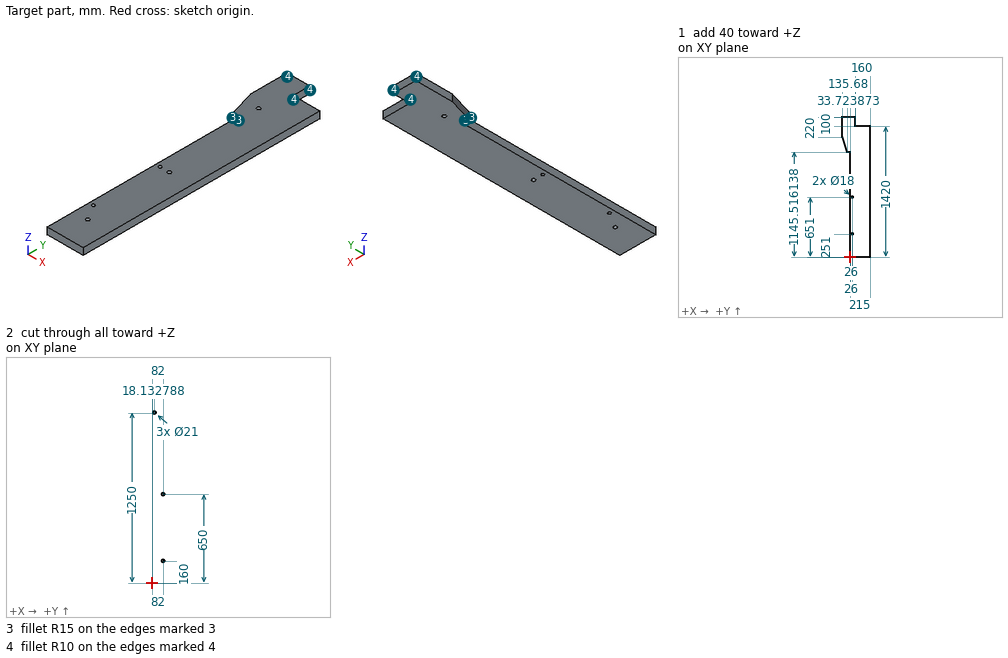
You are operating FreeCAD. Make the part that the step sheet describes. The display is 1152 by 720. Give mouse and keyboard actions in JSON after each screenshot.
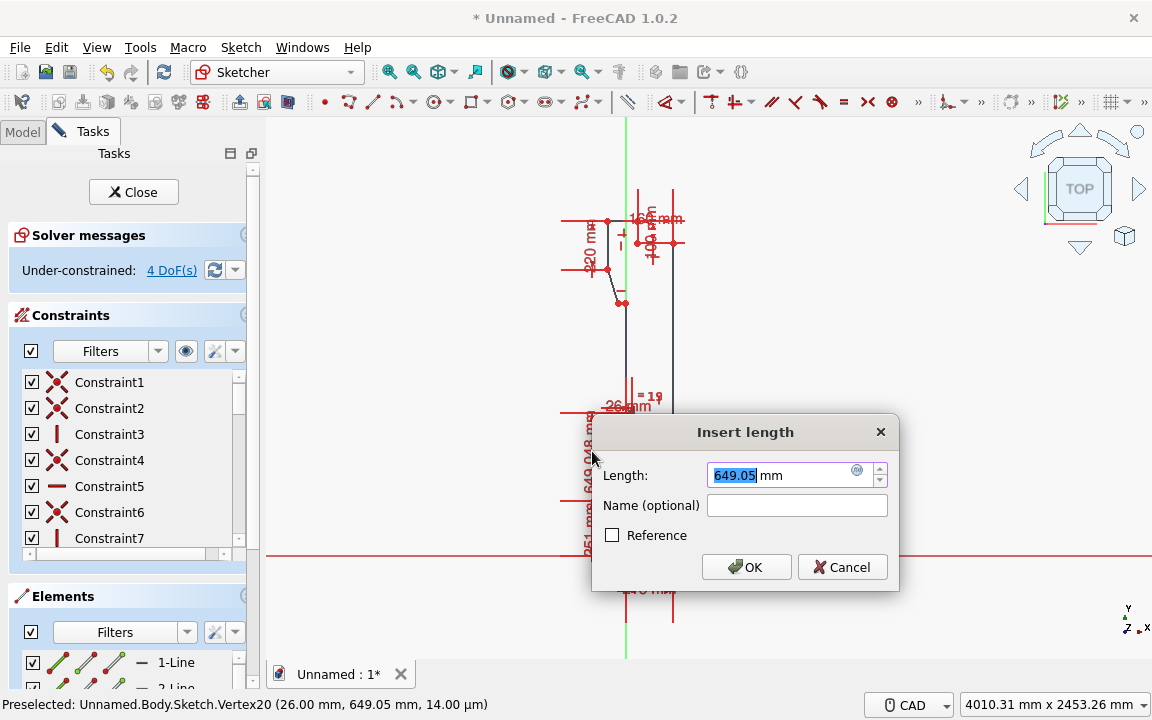
{"action": "type", "text": "651"}
{"action": "key", "text": "Return"}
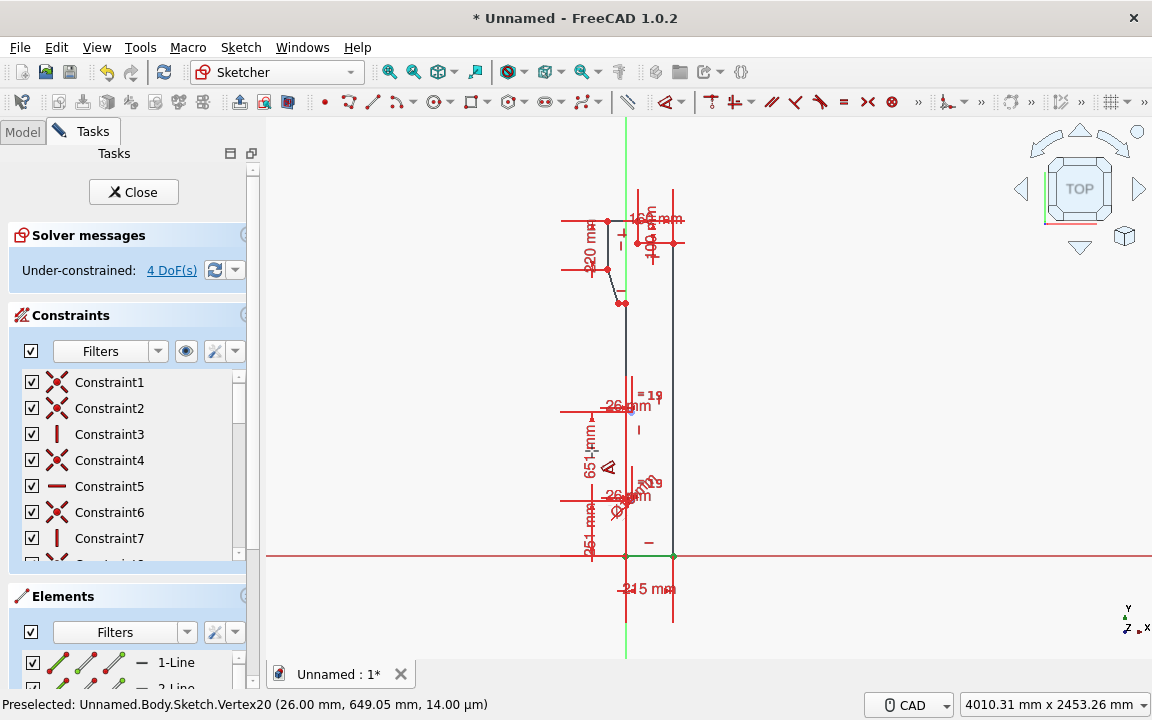
{"action": "left_click", "coordinate": [673, 462]}
{"action": "left_click", "coordinate": [707, 400]}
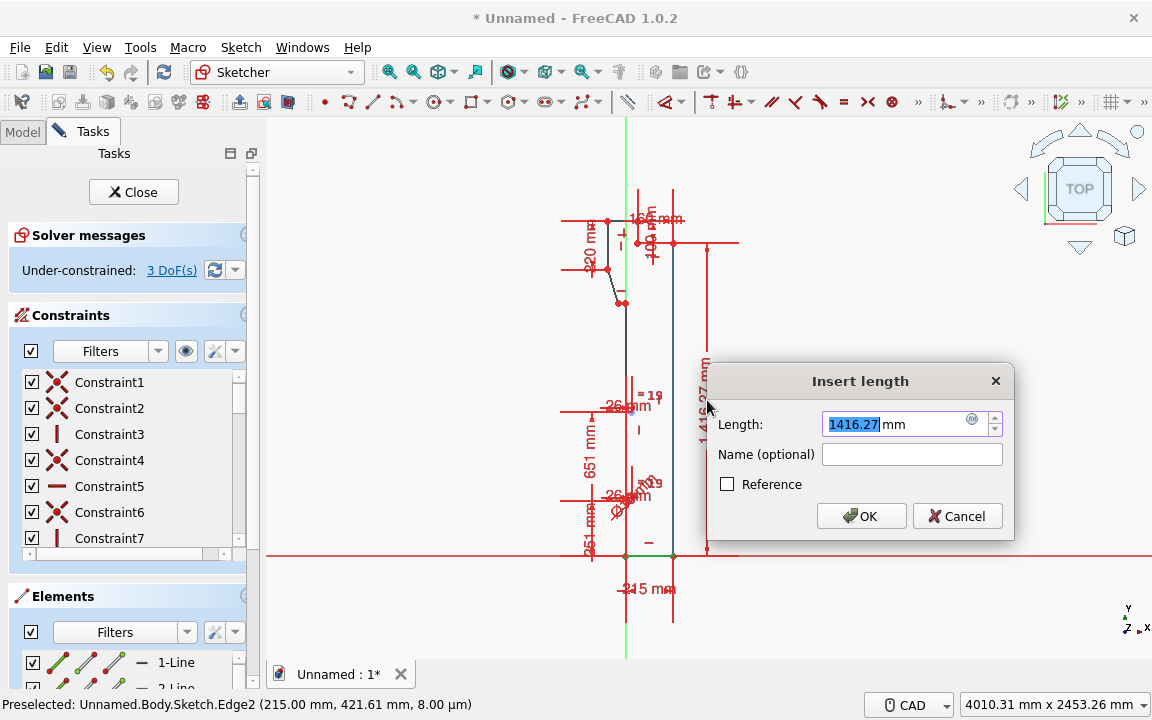
{"action": "type", "text": "1420"}
{"action": "key", "text": "Return"}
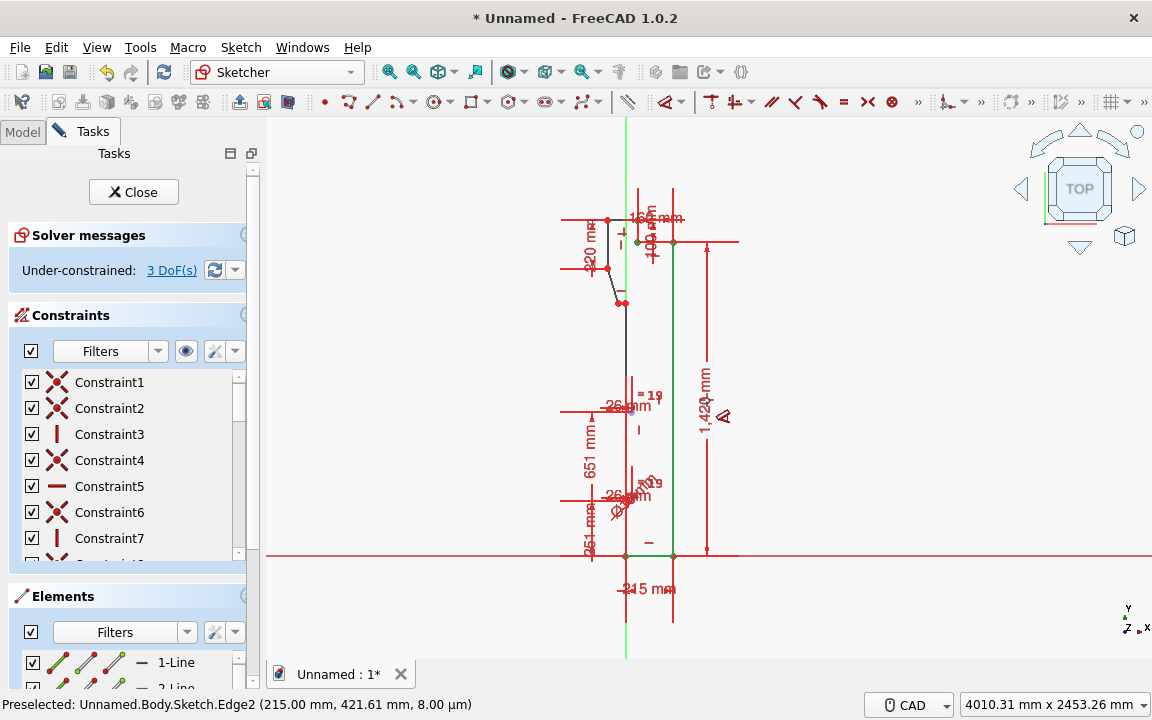
{"action": "scroll", "coordinate": [629, 220], "scroll_direction": "up", "scroll_amount": 3}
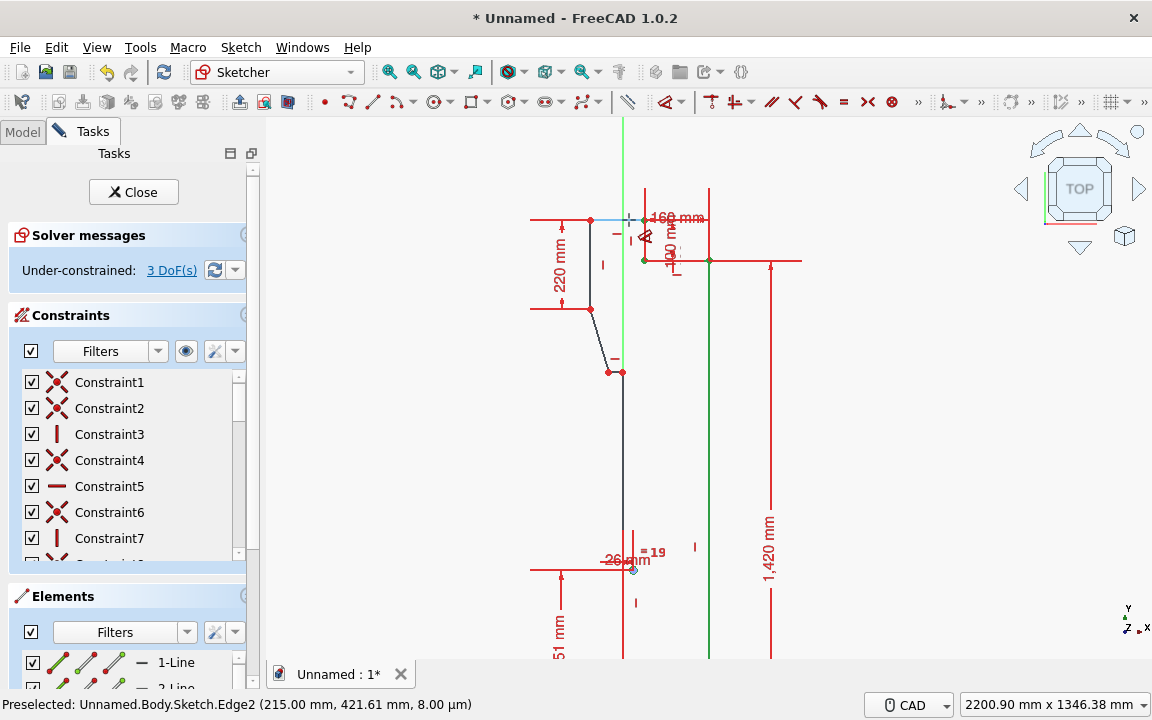
{"action": "left_click", "coordinate": [628, 220]}
{"action": "left_click", "coordinate": [605, 186]}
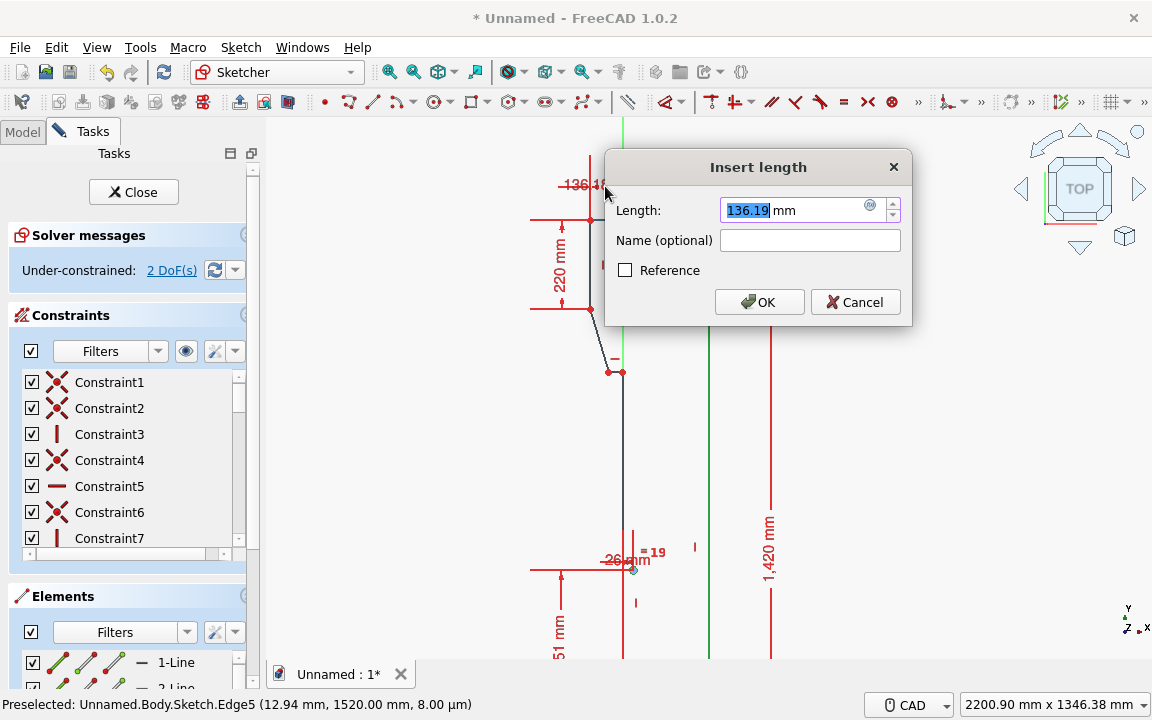
{"action": "type", "text": "135.68"}
{"action": "key", "text": "Return"}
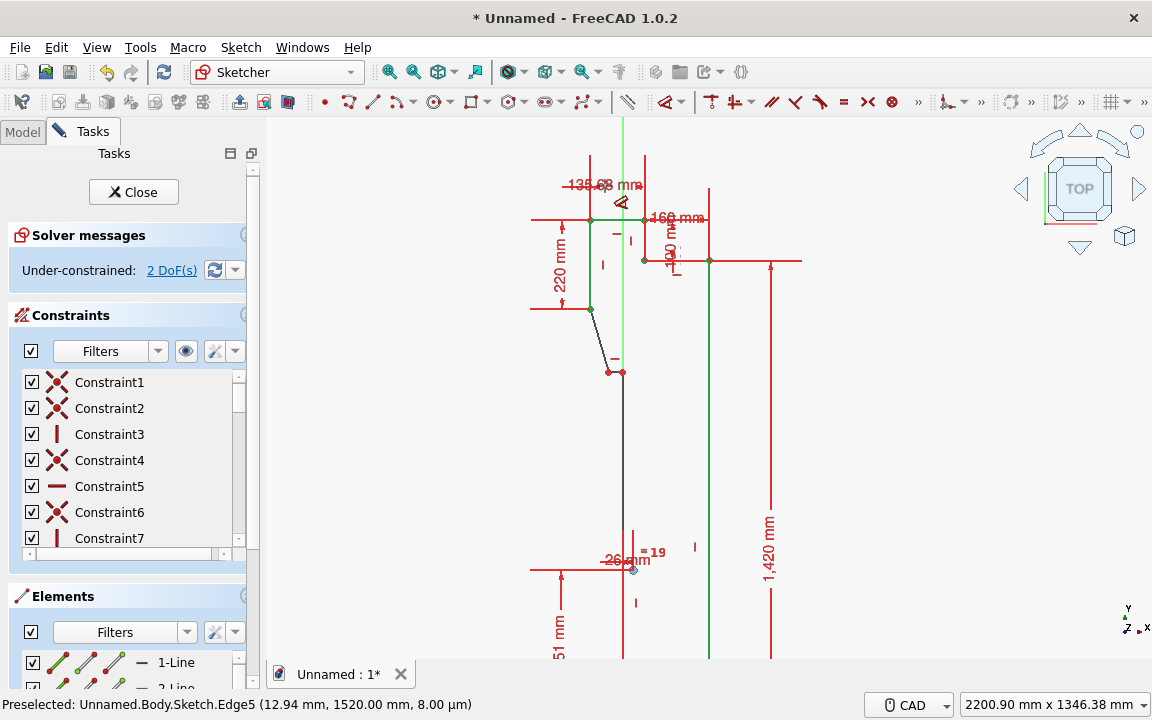
{"action": "scroll", "coordinate": [616, 372], "scroll_direction": "up", "scroll_amount": 6}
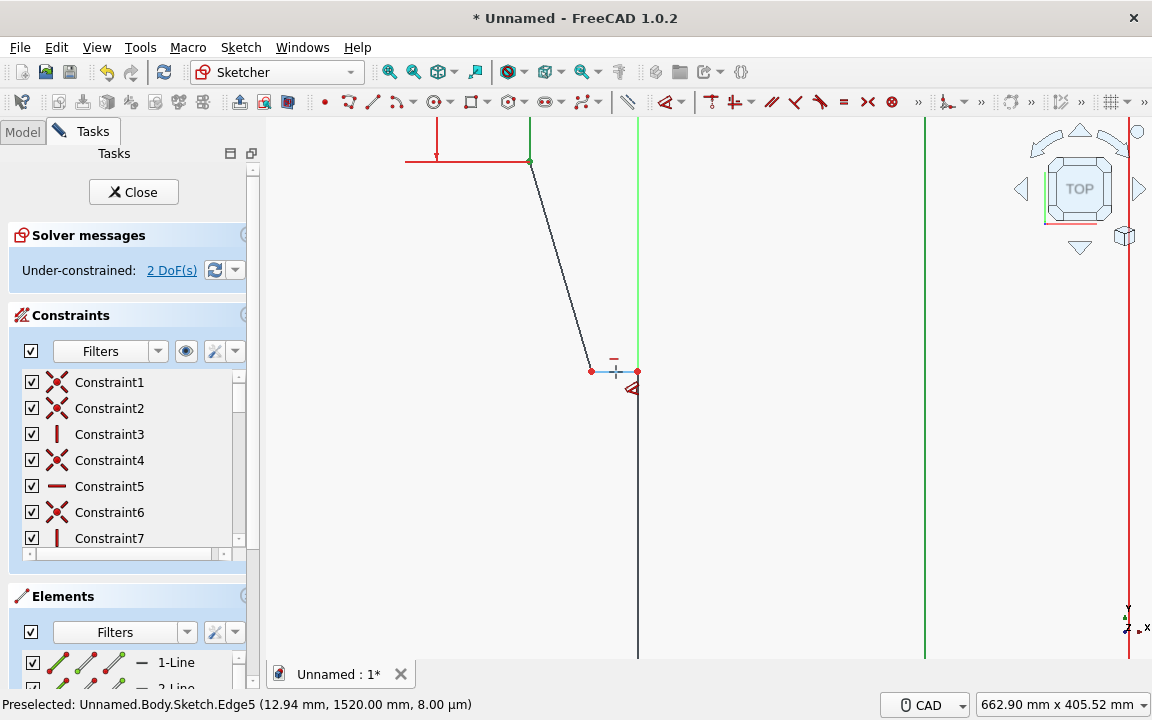
{"action": "left_click", "coordinate": [615, 372]}
{"action": "left_click", "coordinate": [615, 338]}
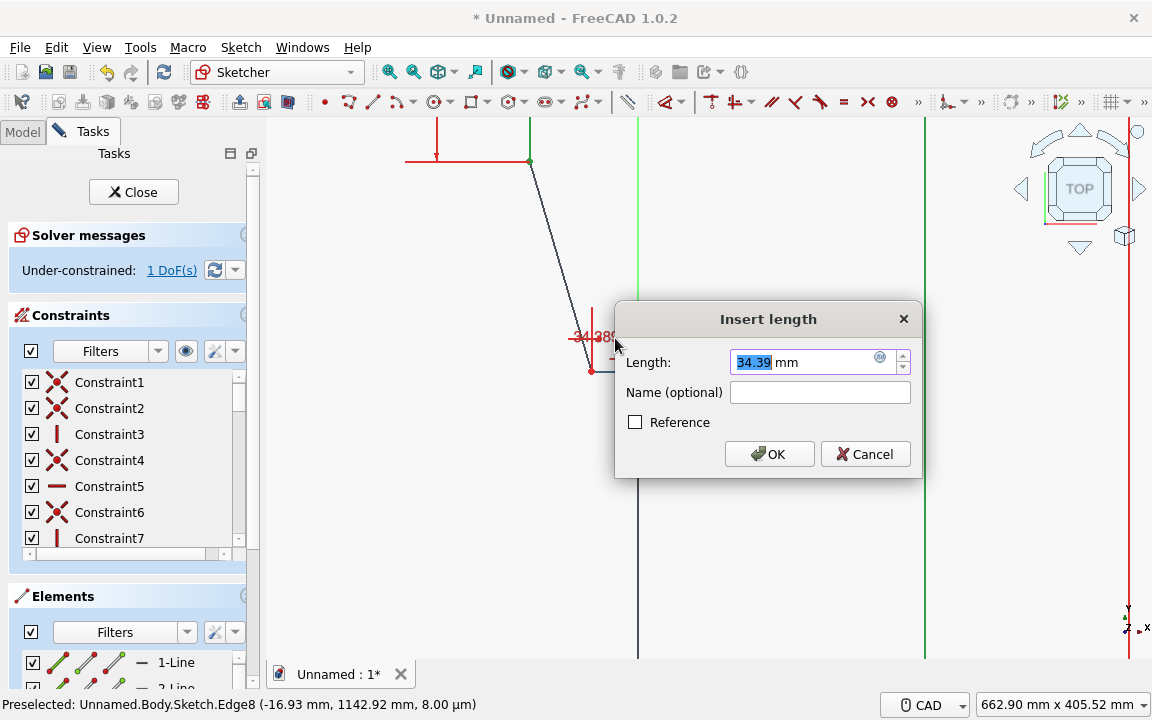
{"action": "type", "text": "33.723873"}
{"action": "key", "text": "Return"}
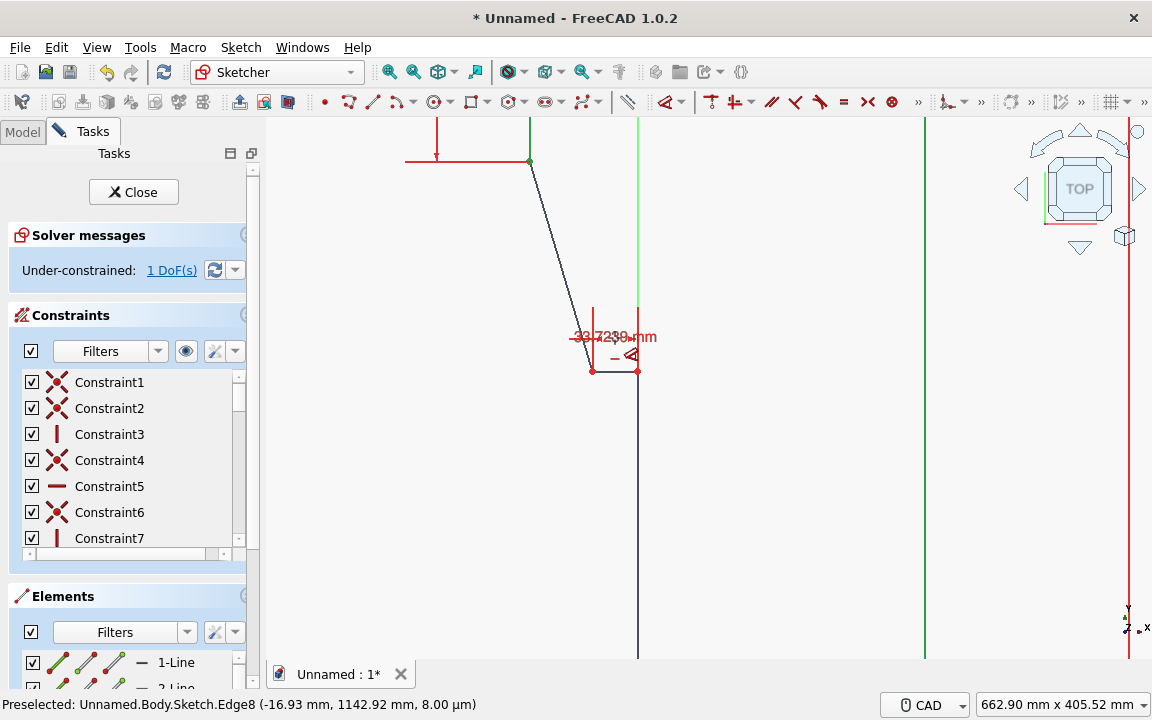
{"action": "scroll", "coordinate": [623, 290], "scroll_direction": "down", "scroll_amount": 9}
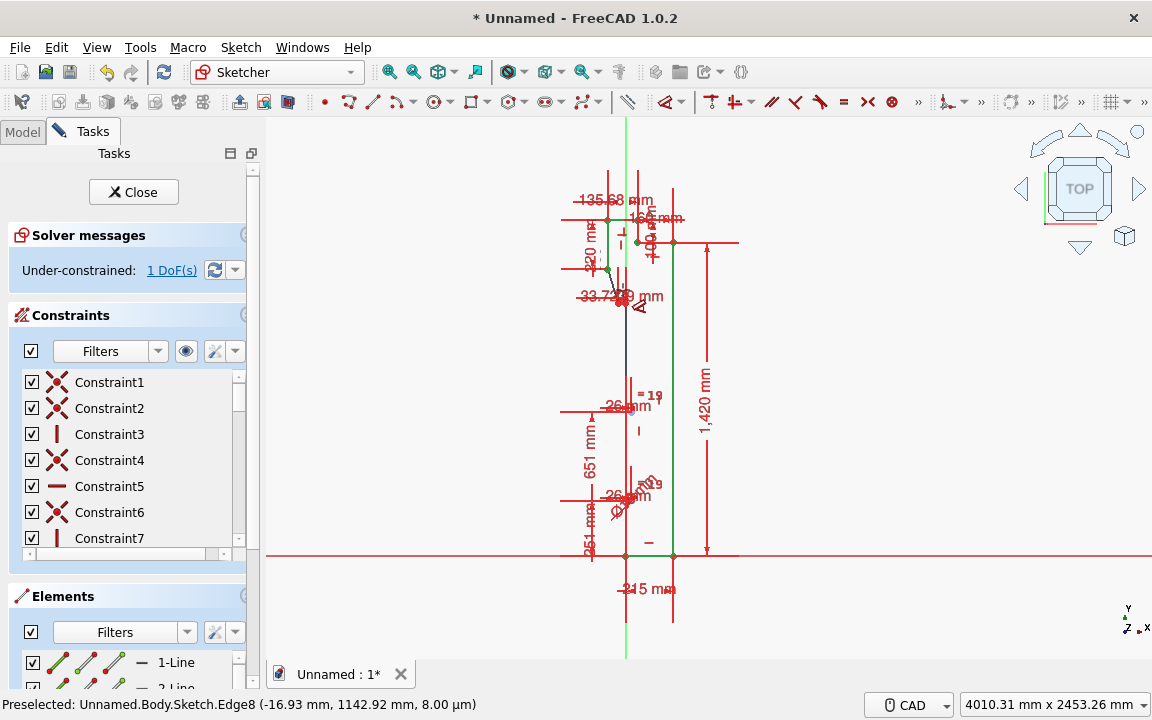
{"action": "left_click", "coordinate": [626, 380]}
{"action": "left_click", "coordinate": [592, 430]}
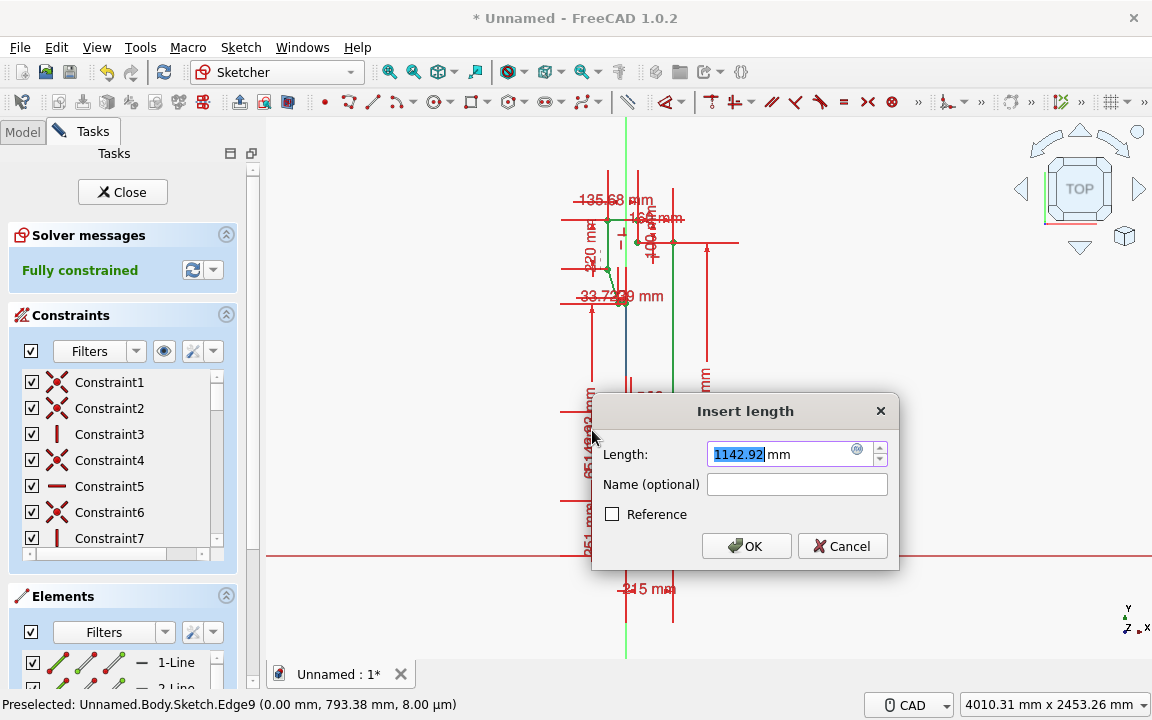
{"action": "type", "text": "1145.516138"}
{"action": "key", "text": "Return"}
{"action": "key", "text": "Escape"}